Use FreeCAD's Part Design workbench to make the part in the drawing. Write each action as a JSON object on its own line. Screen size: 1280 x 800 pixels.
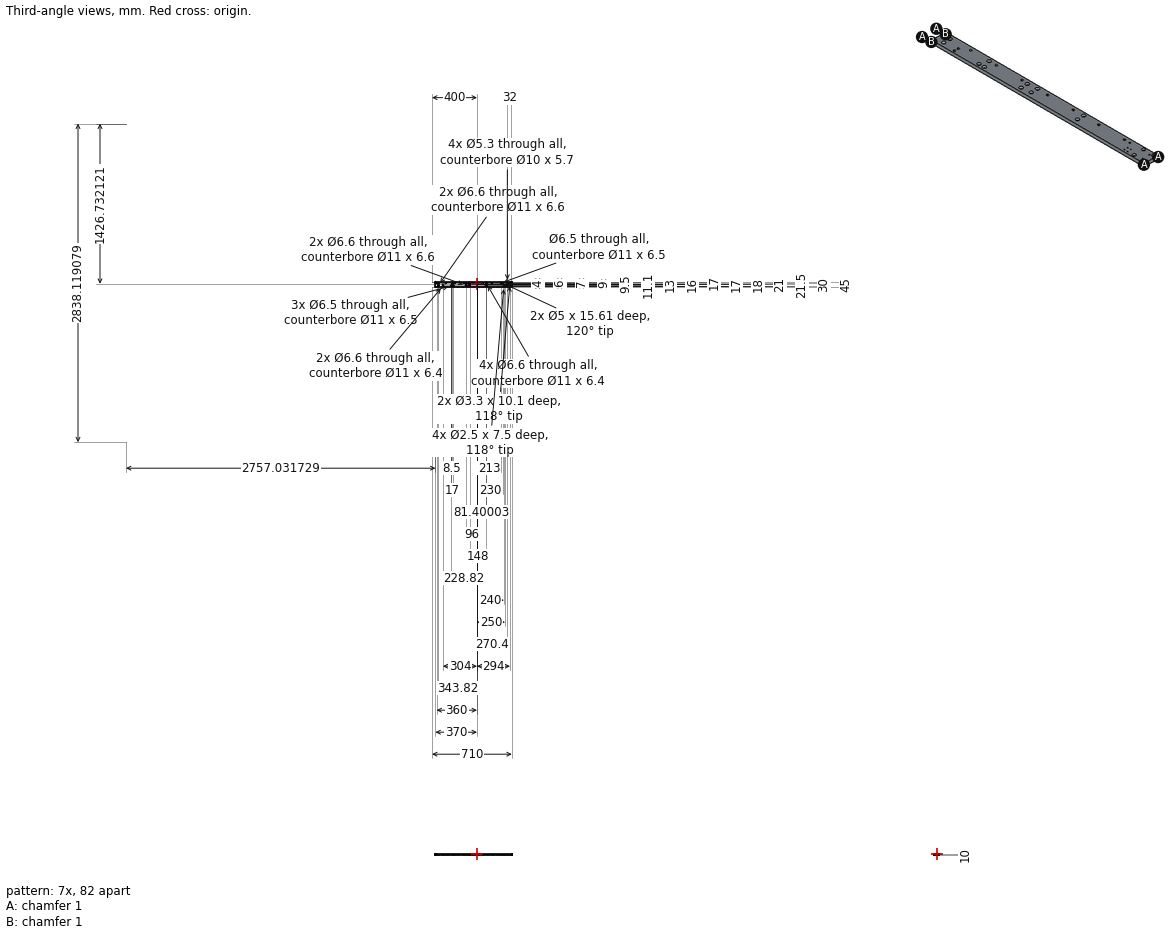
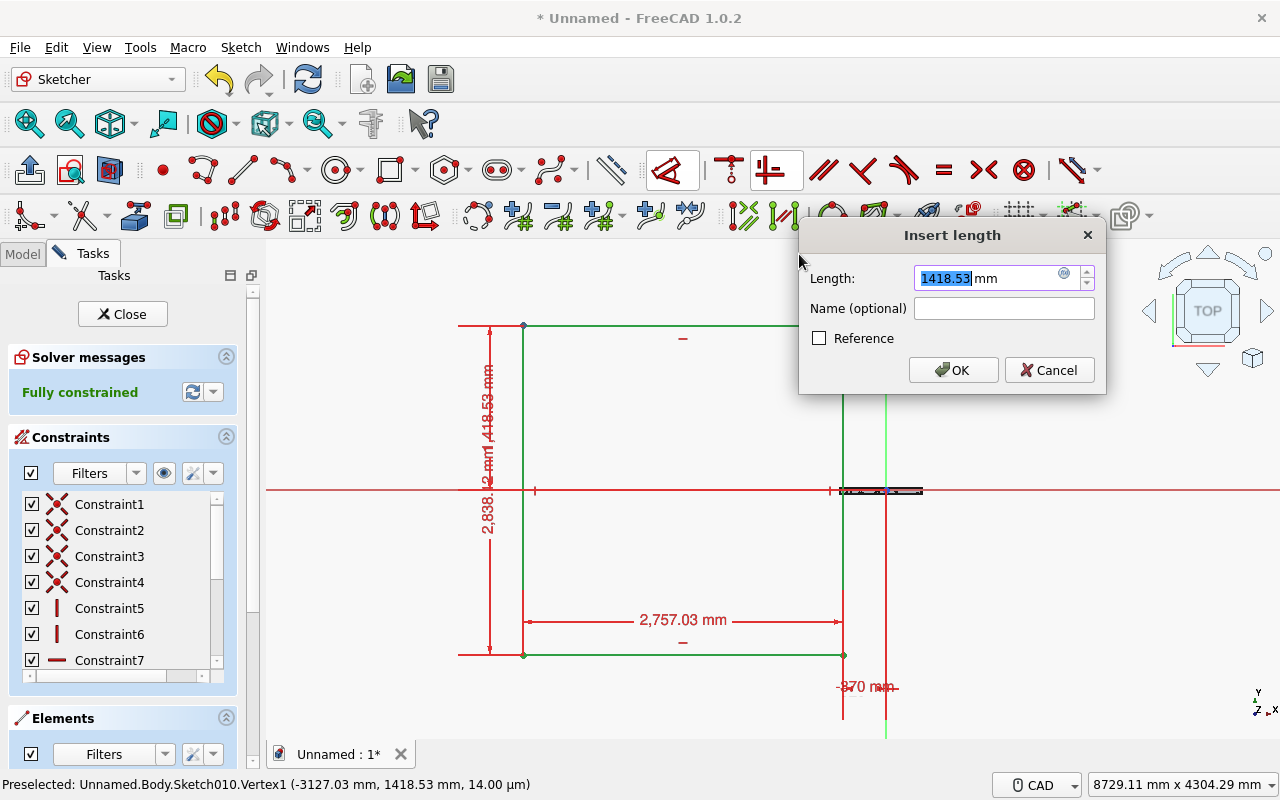
{"action": "type", "text": "1426.732121"}
{"action": "key", "text": "Return"}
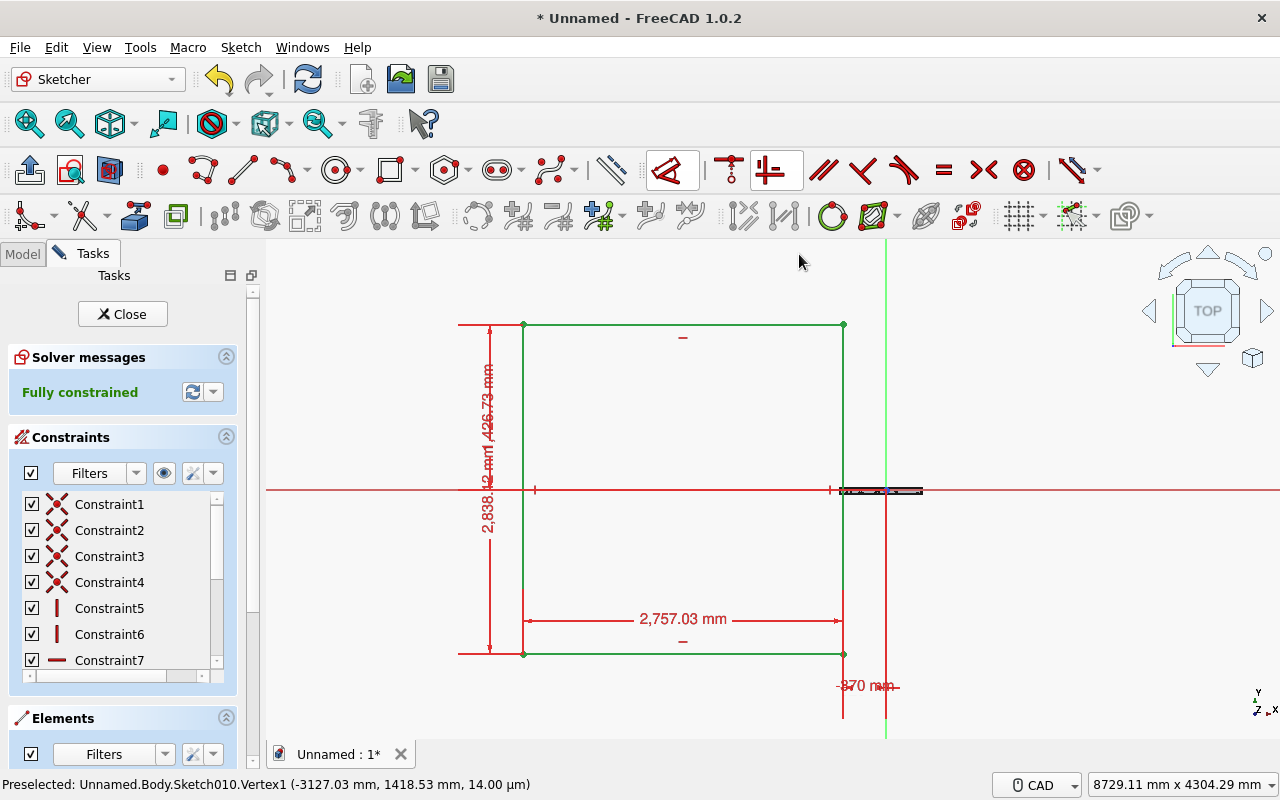
{"action": "left_click", "coordinate": [123, 314]}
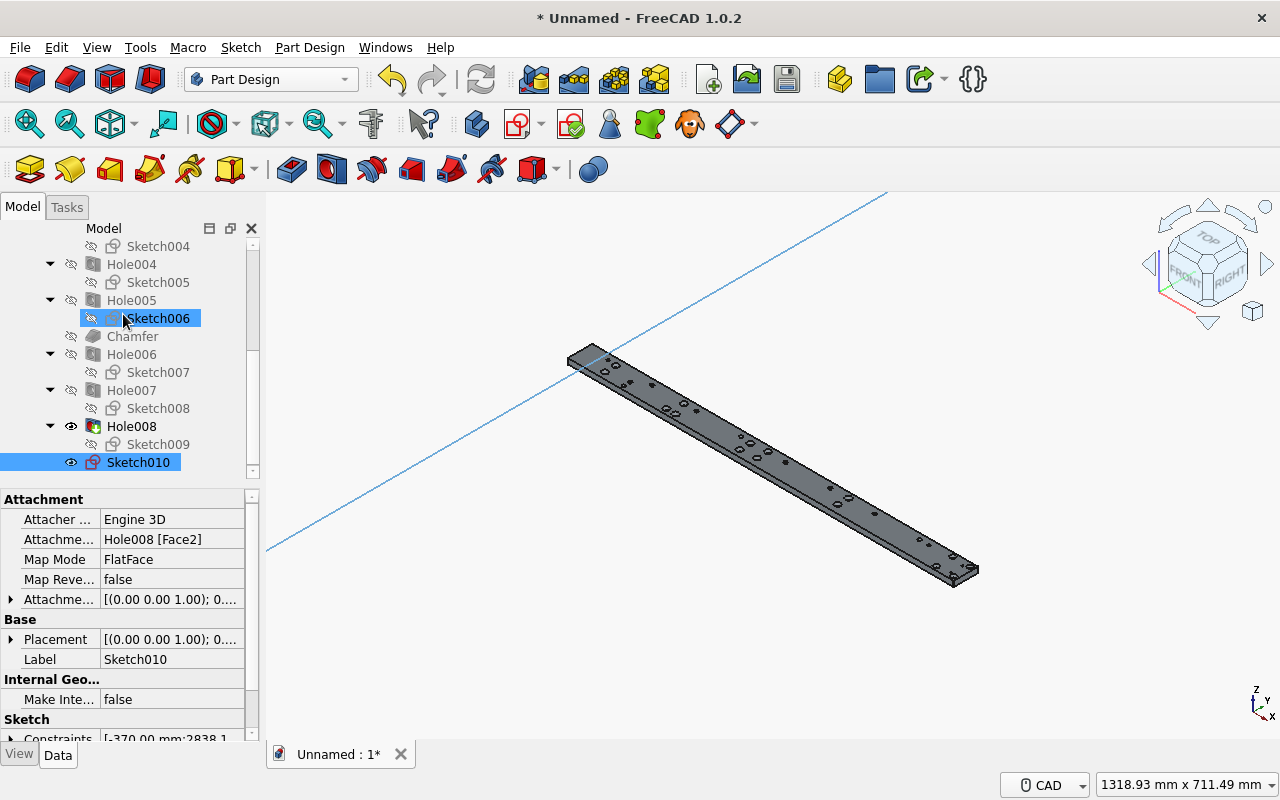
{"action": "left_click", "coordinate": [292, 170]}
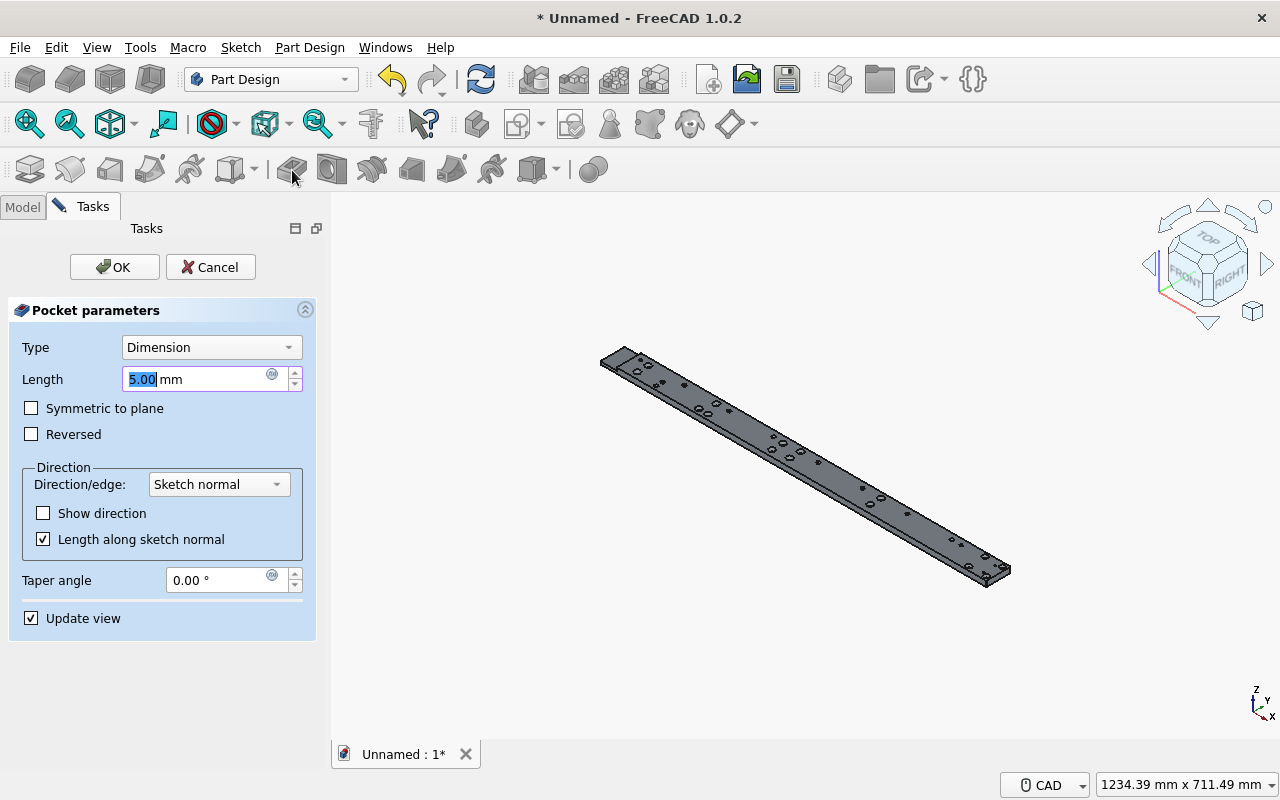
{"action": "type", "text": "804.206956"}
{"action": "key", "text": "Tab"}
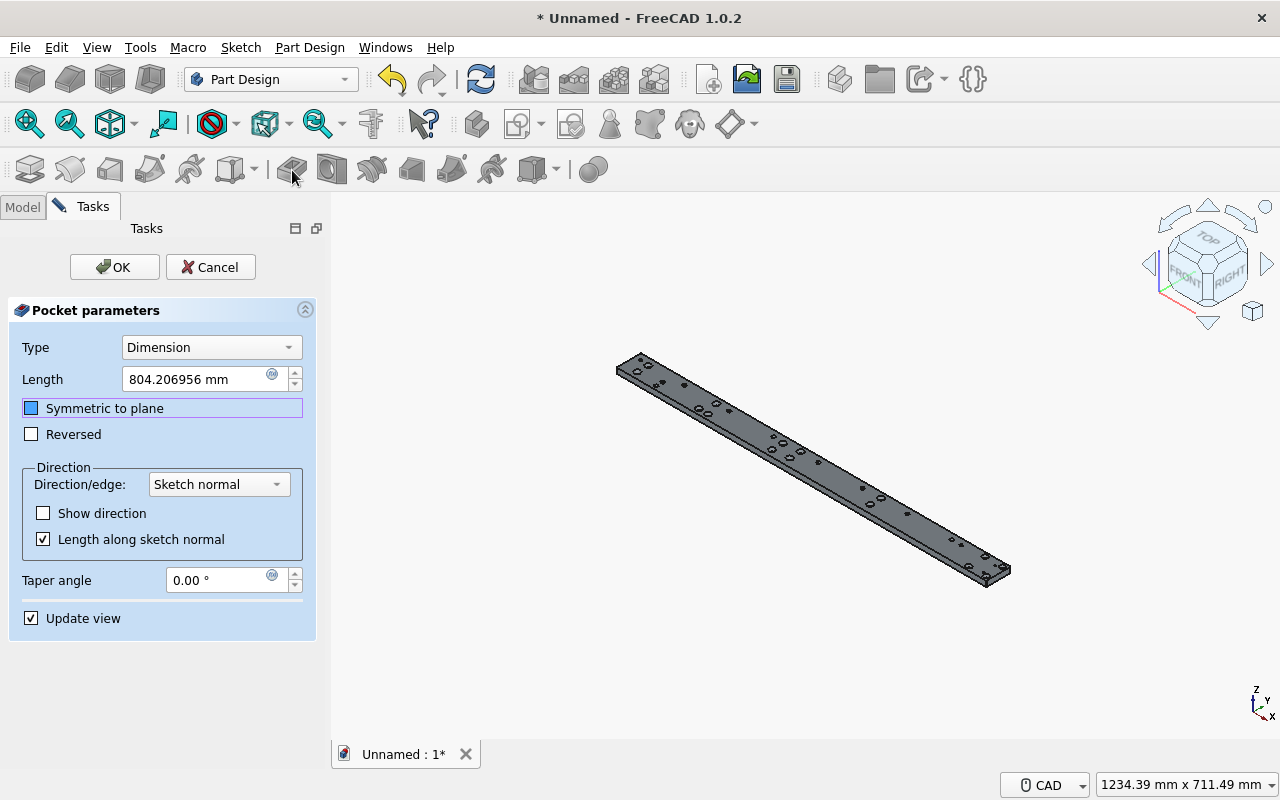
{"action": "left_click", "coordinate": [30, 408]}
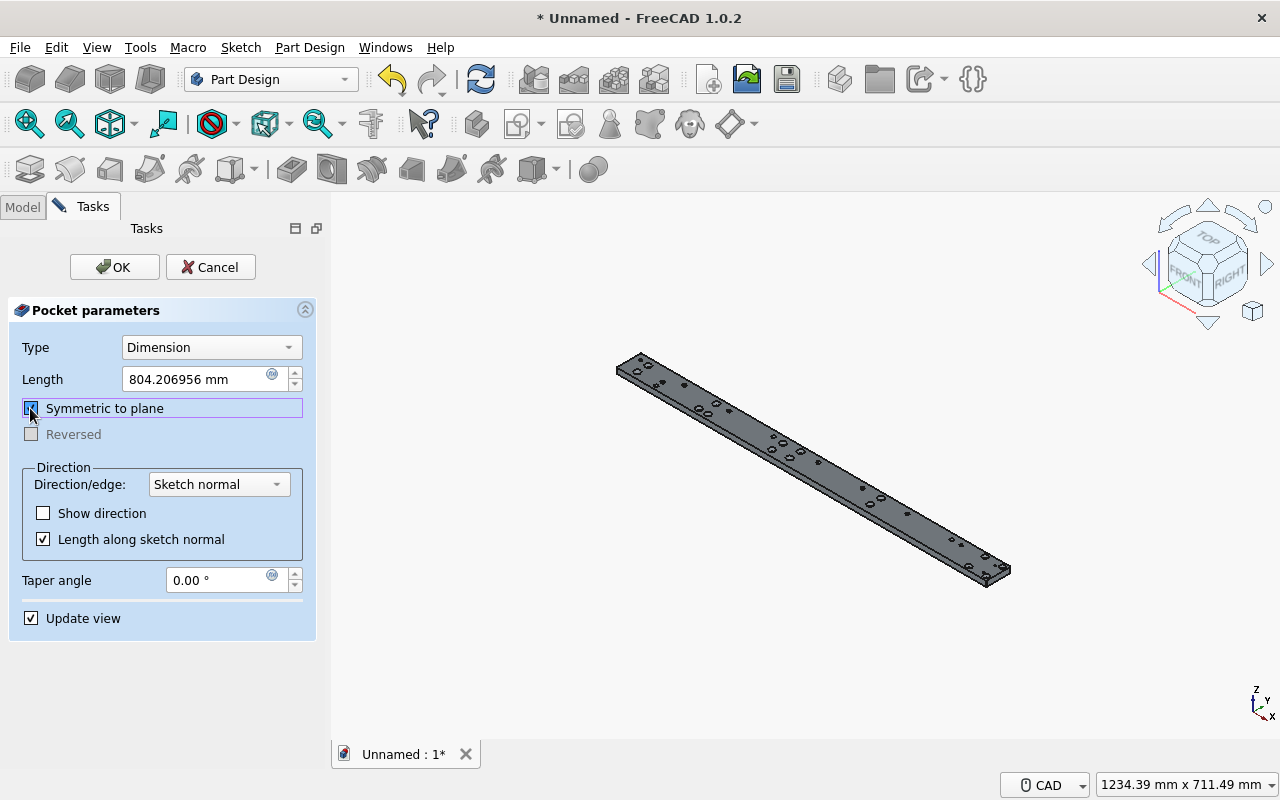
{"action": "left_click", "coordinate": [115, 267]}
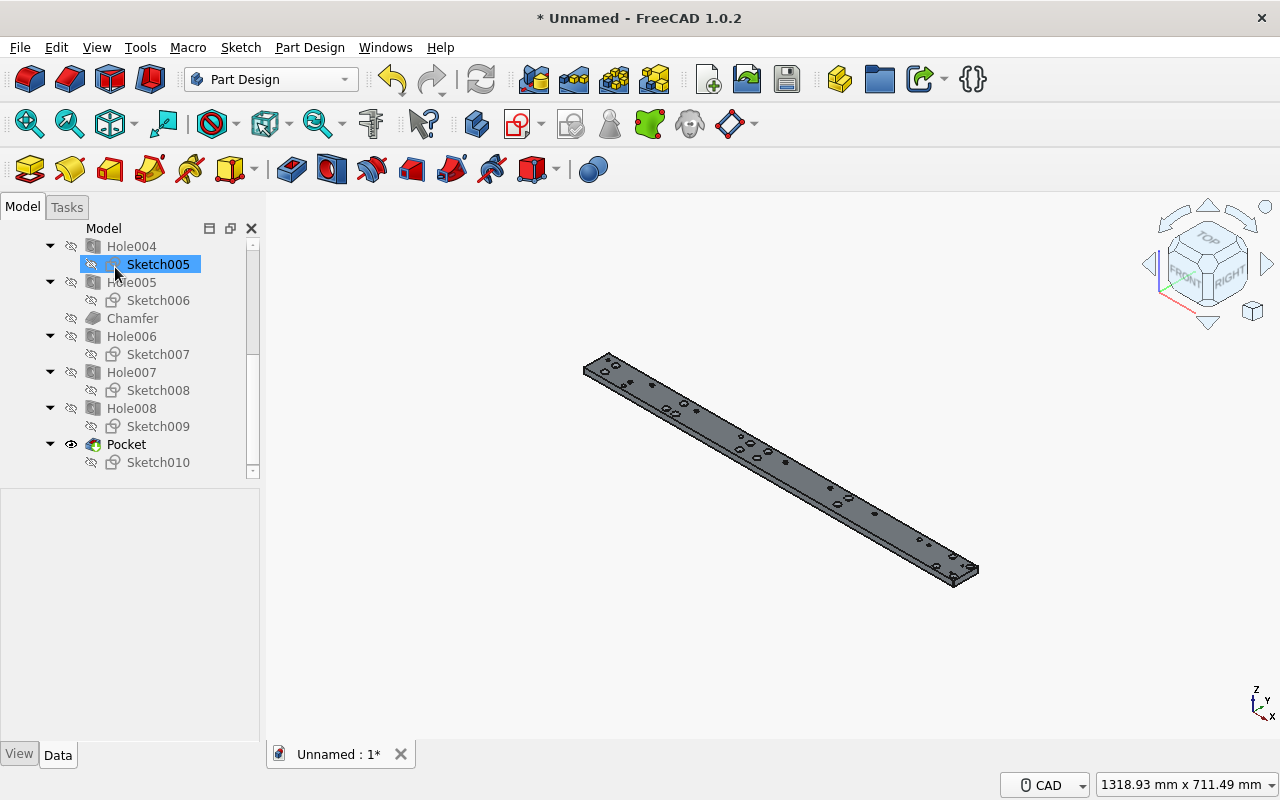
{"action": "left_click", "coordinate": [30, 124]}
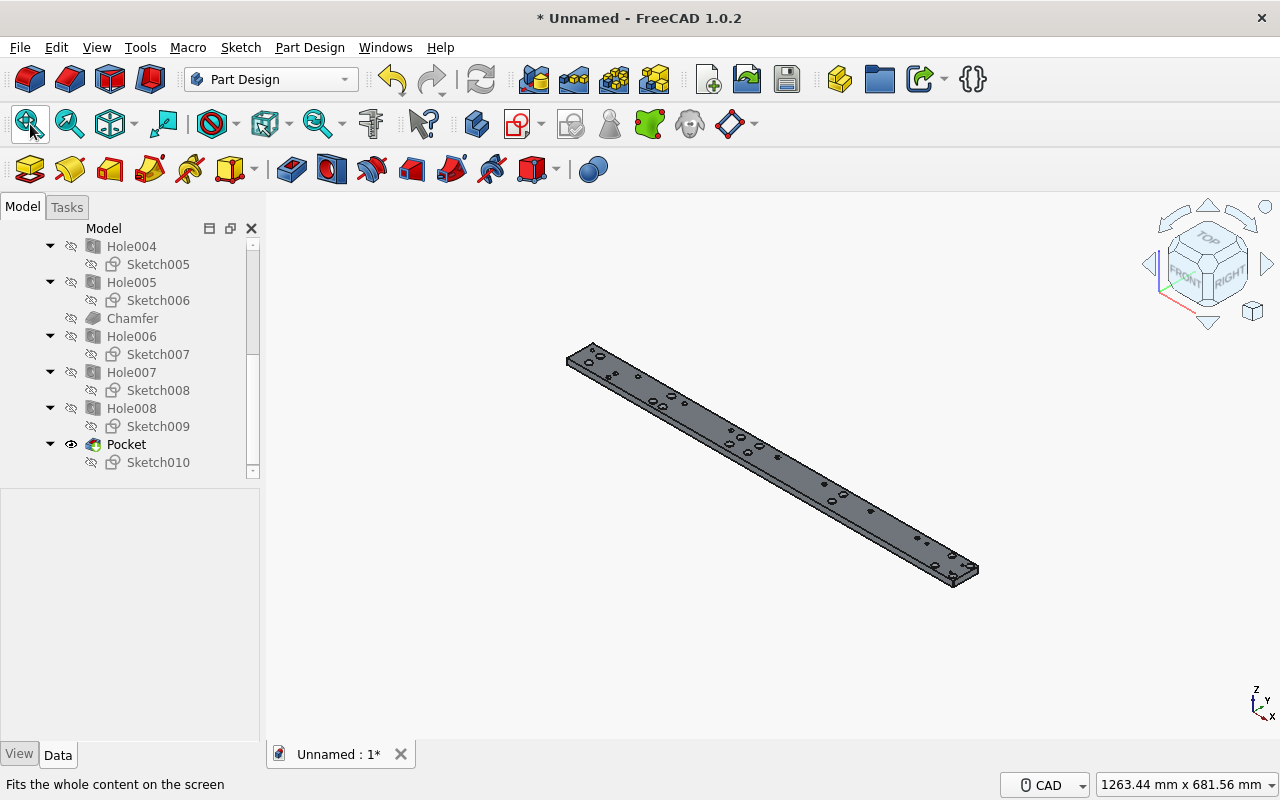
{"action": "scroll", "coordinate": [567, 360], "scroll_direction": "up", "scroll_amount": 9}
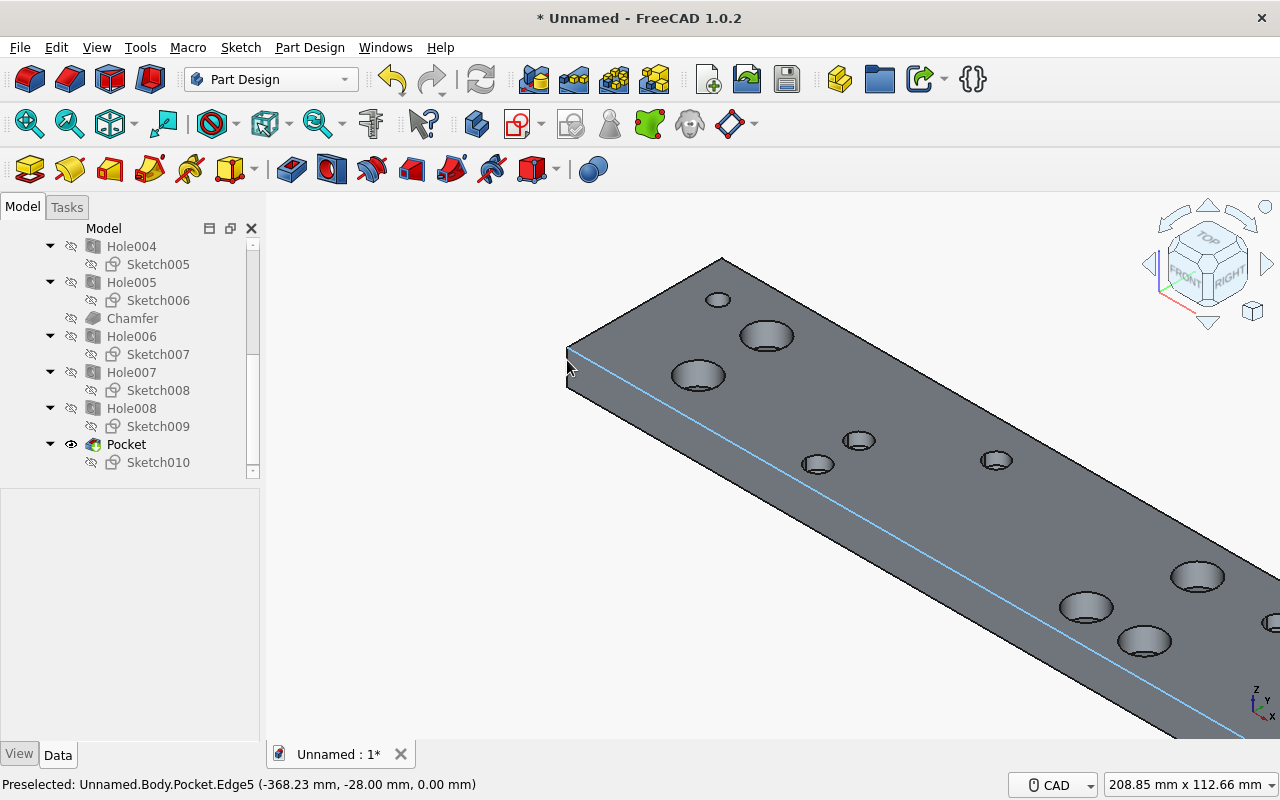
{"action": "left_click", "coordinate": [30, 124]}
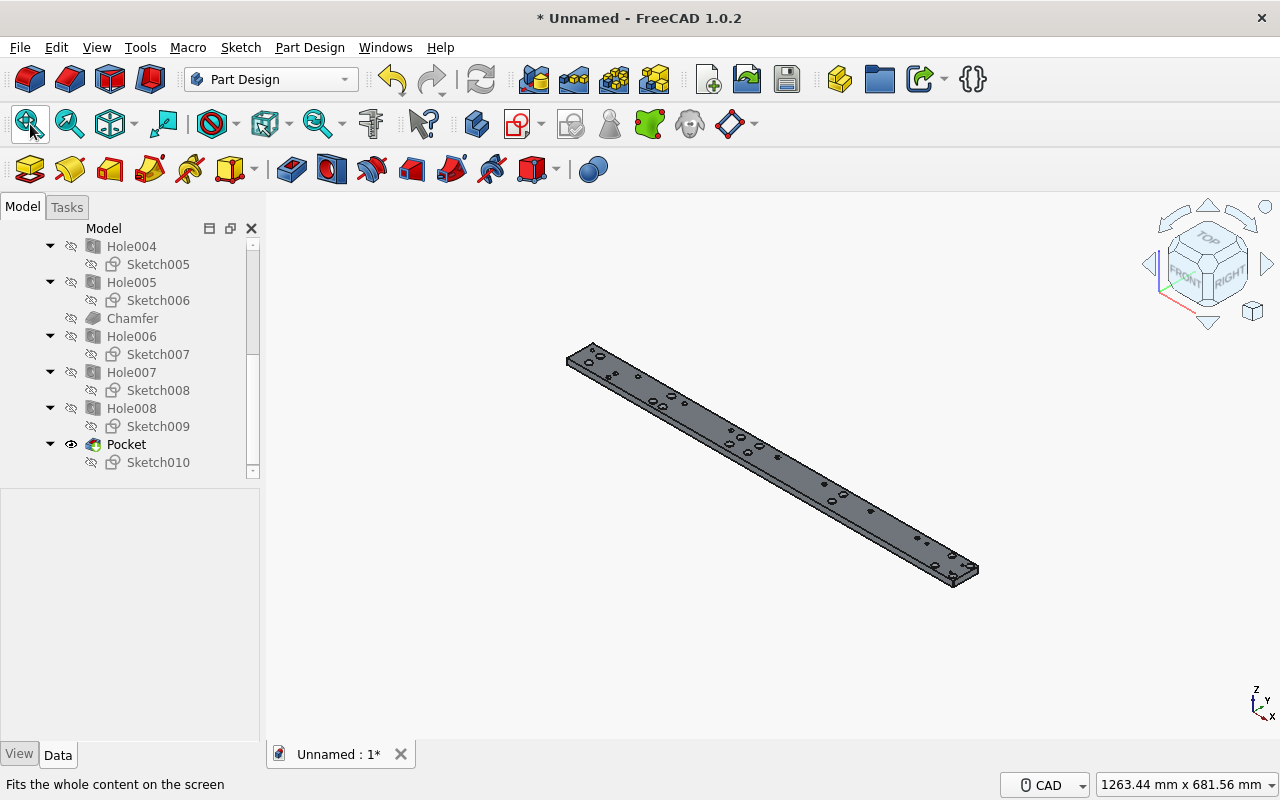
{"action": "key", "text": "2"}